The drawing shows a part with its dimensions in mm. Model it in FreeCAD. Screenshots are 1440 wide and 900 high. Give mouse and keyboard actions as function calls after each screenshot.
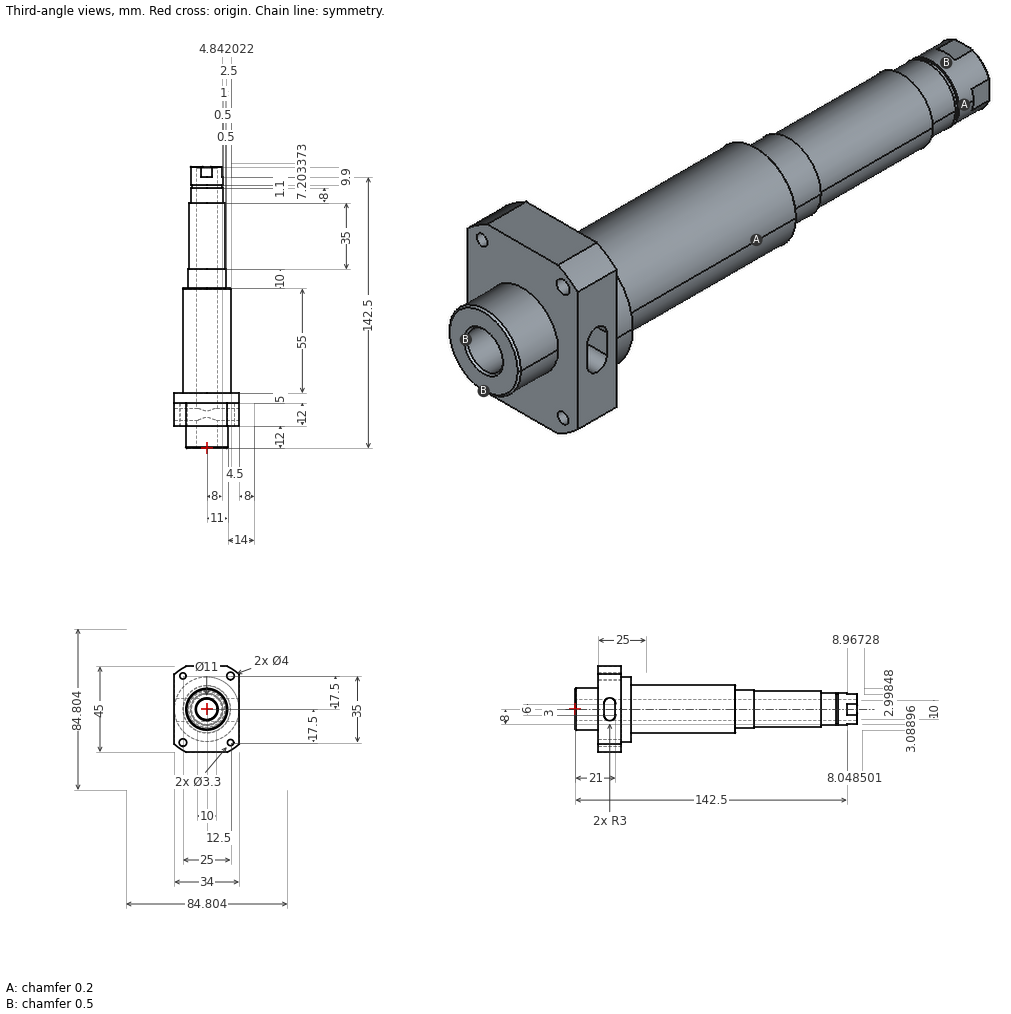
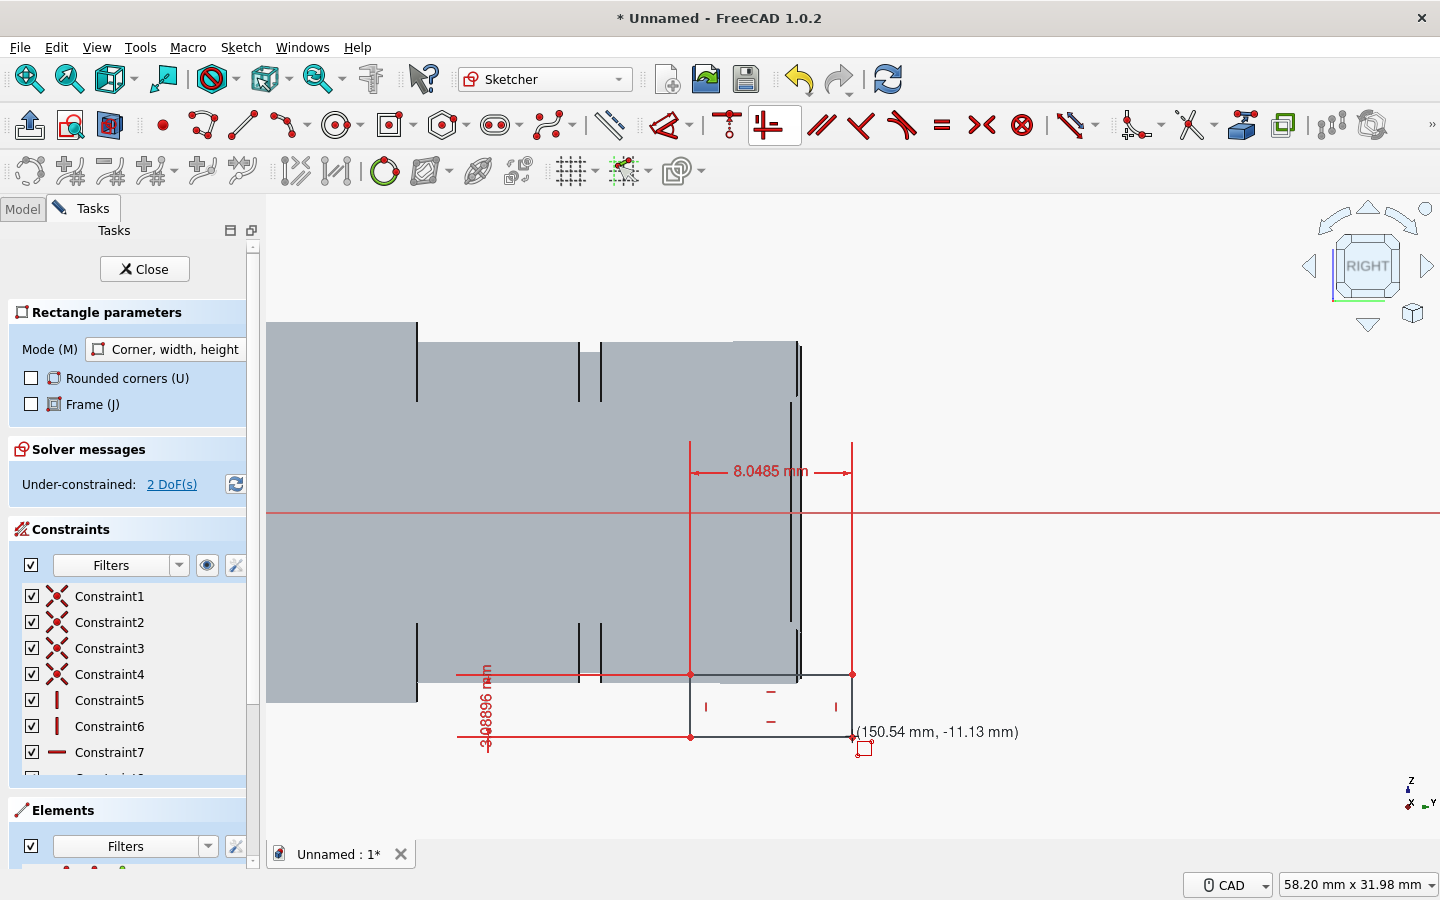
click(690, 291)
move(871, 351)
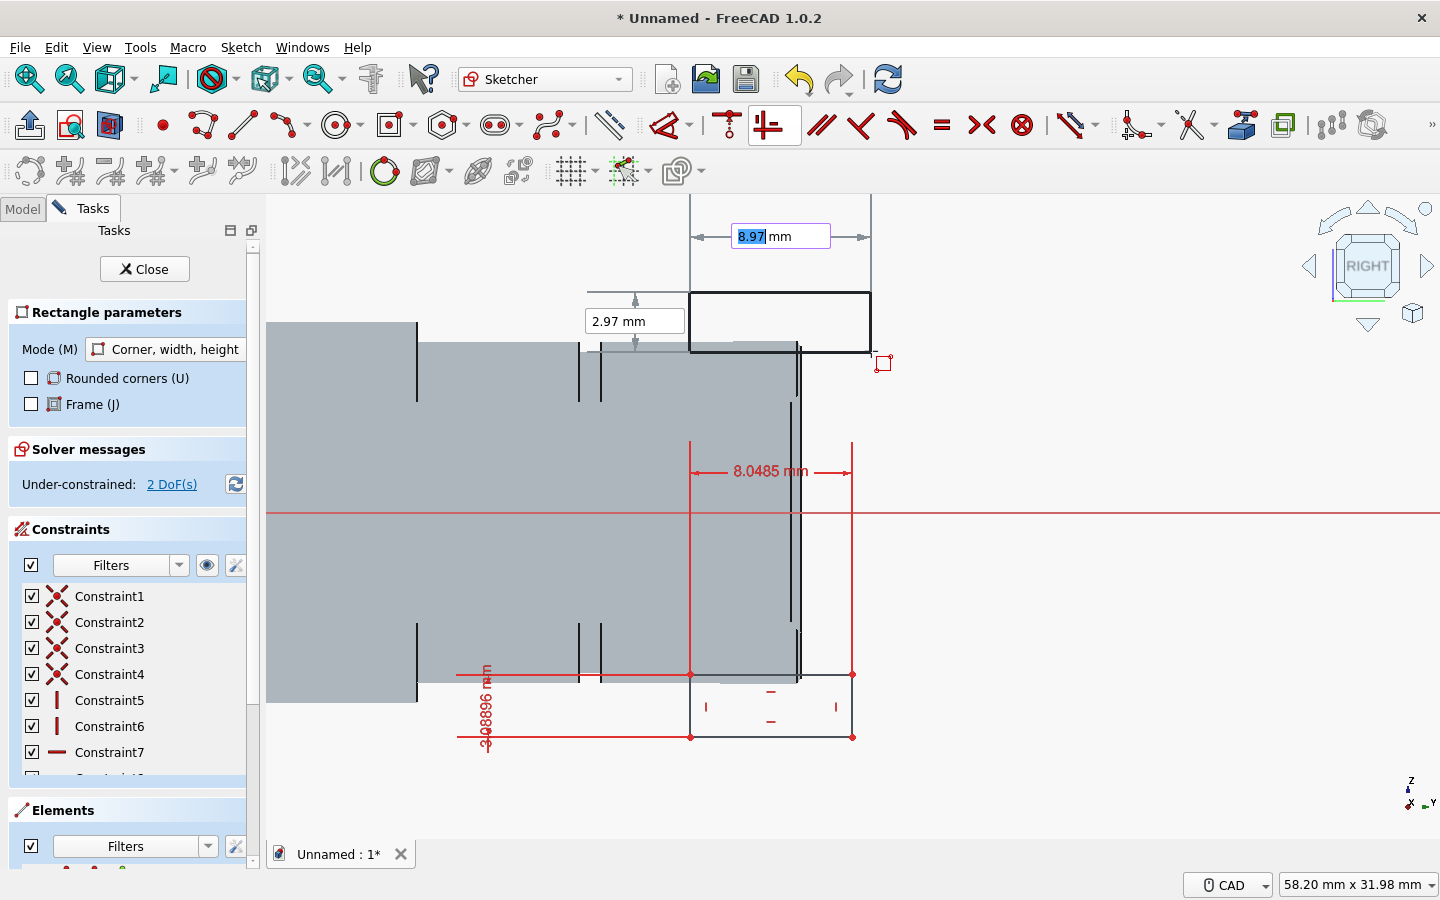
text(8.96728)
key(Tab)
text(2.99848)
key(Return)
key(Escape)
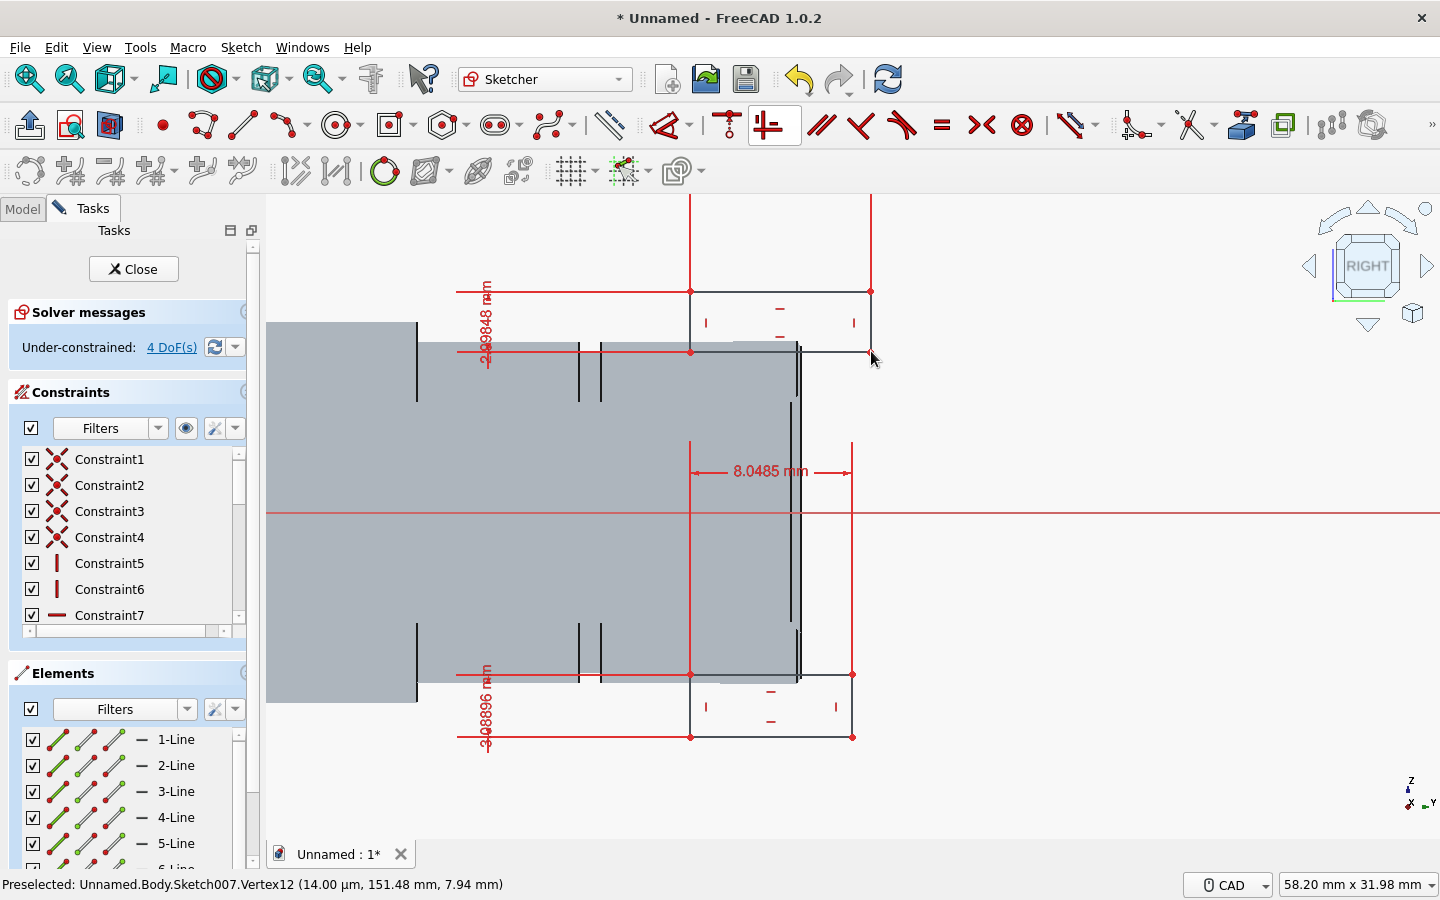
click(690, 675)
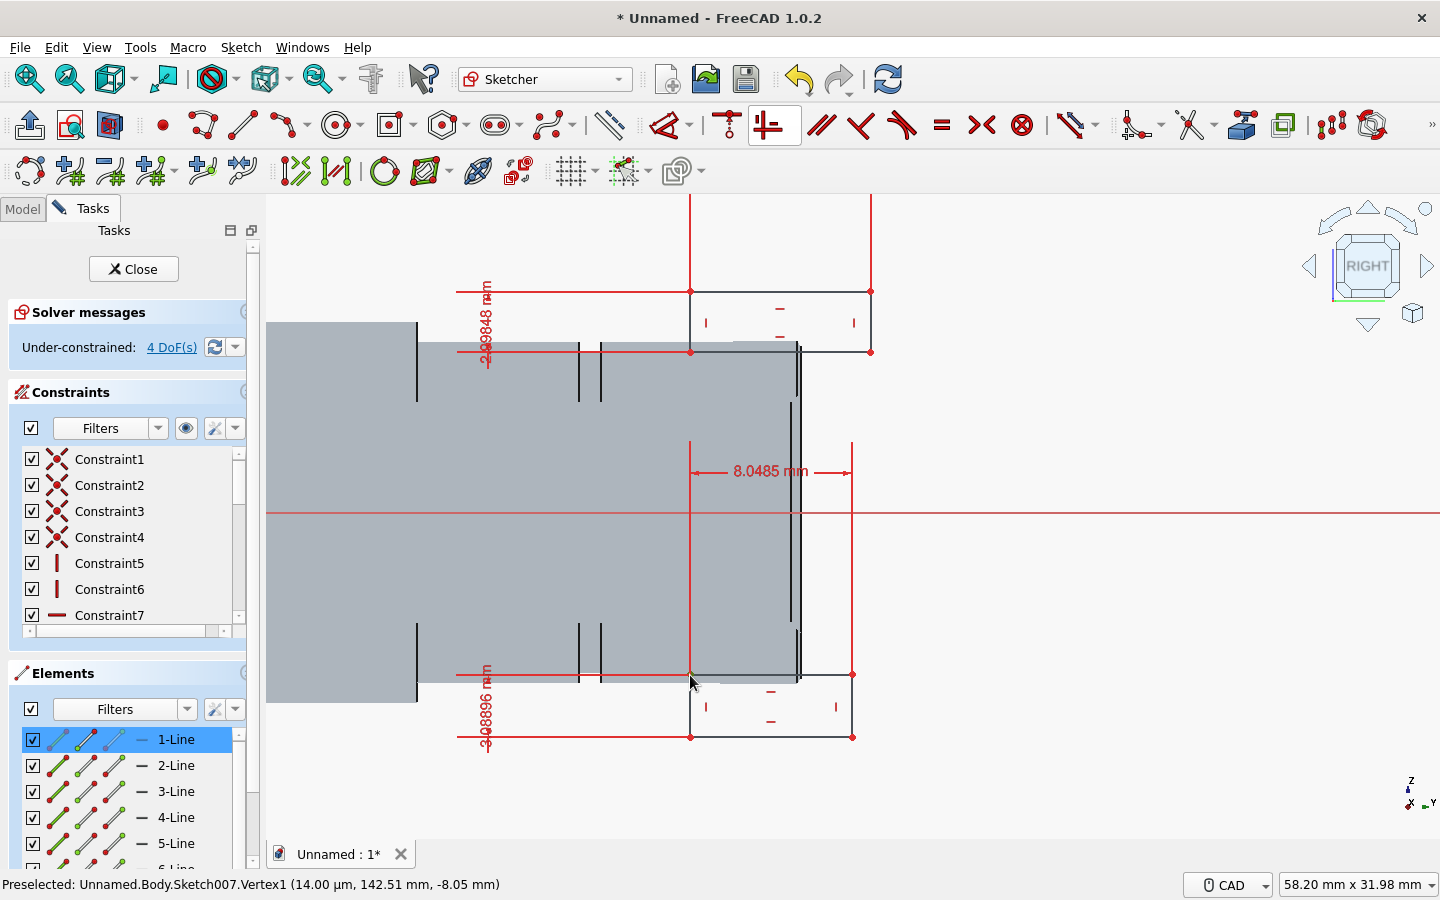
click(690, 352)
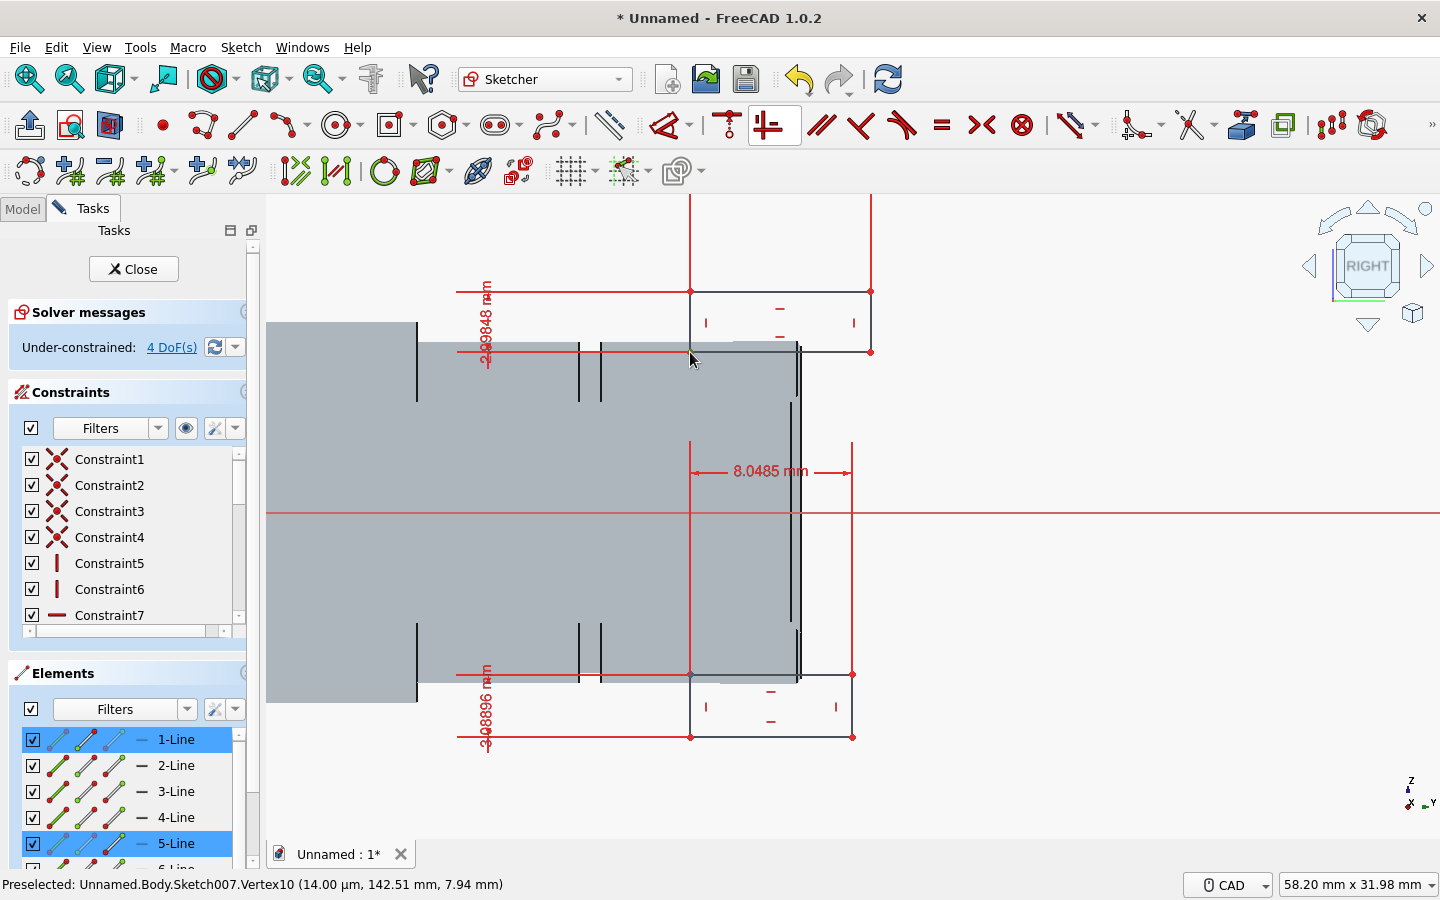
click(364, 513)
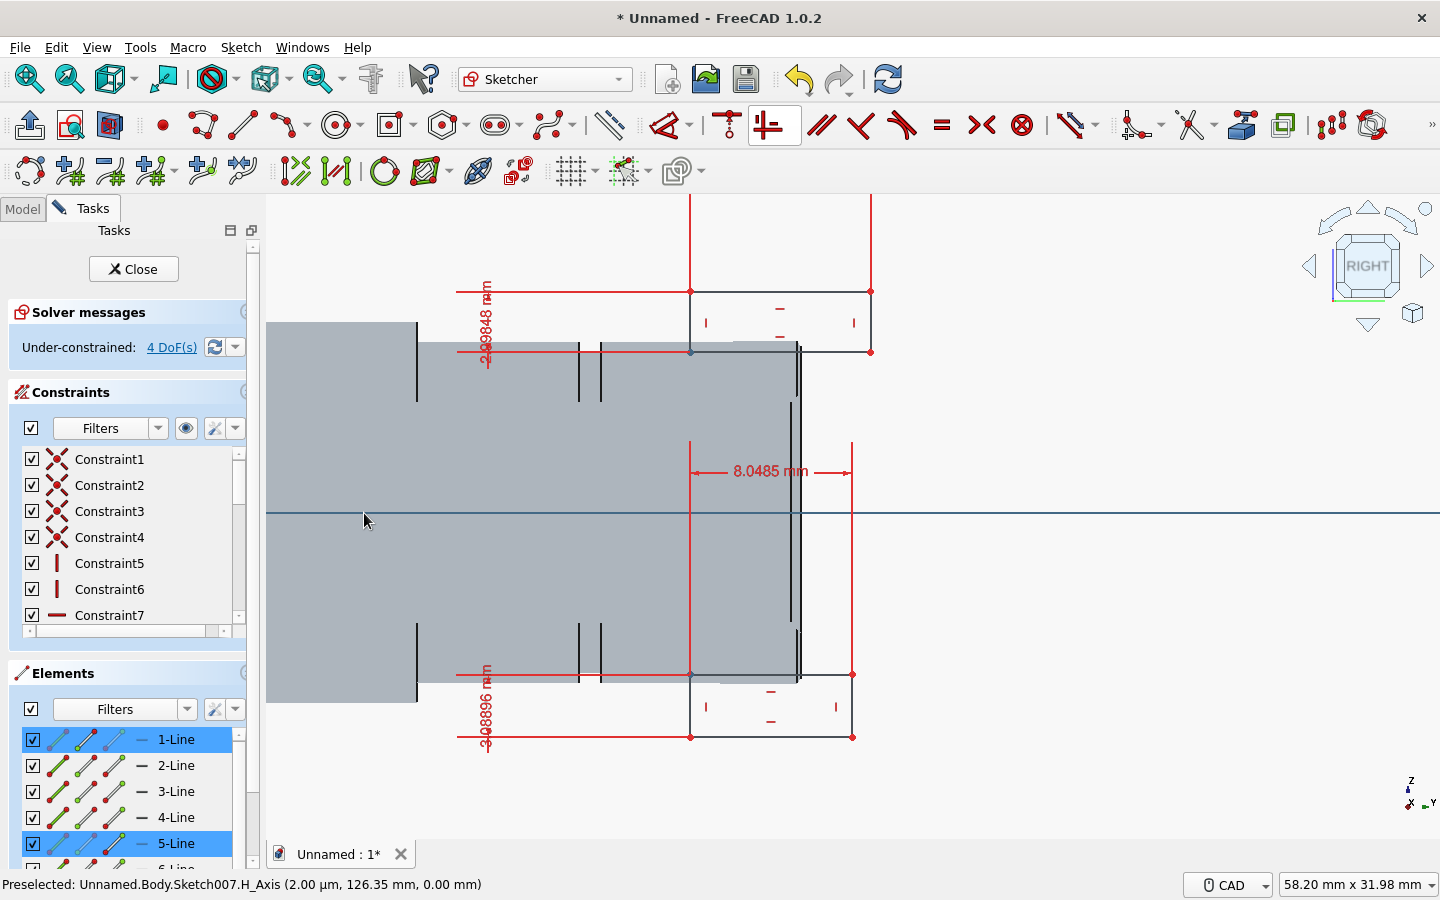
click(982, 126)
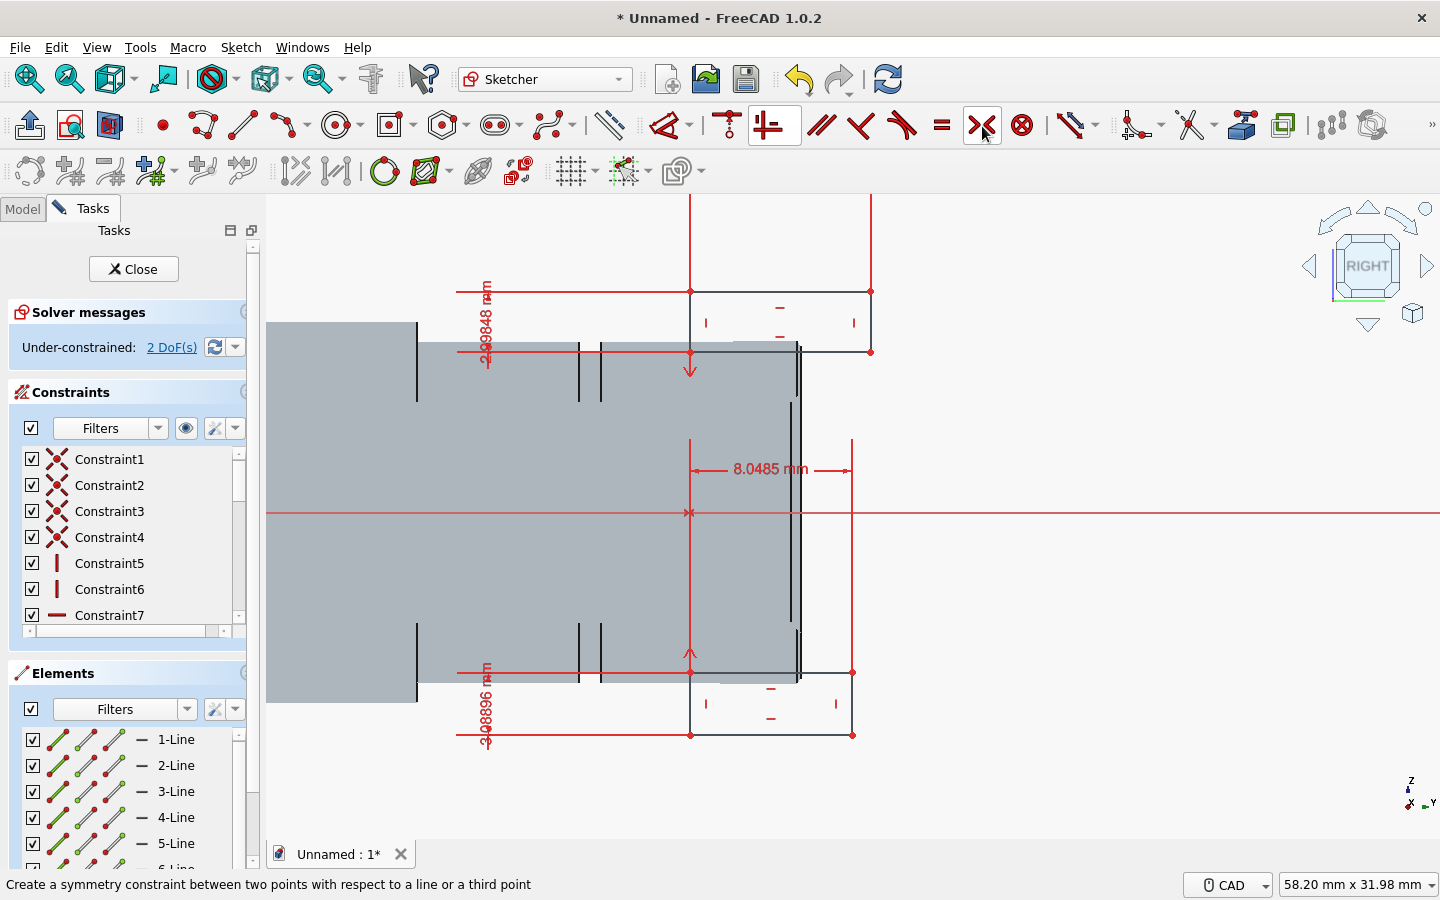
click(664, 126)